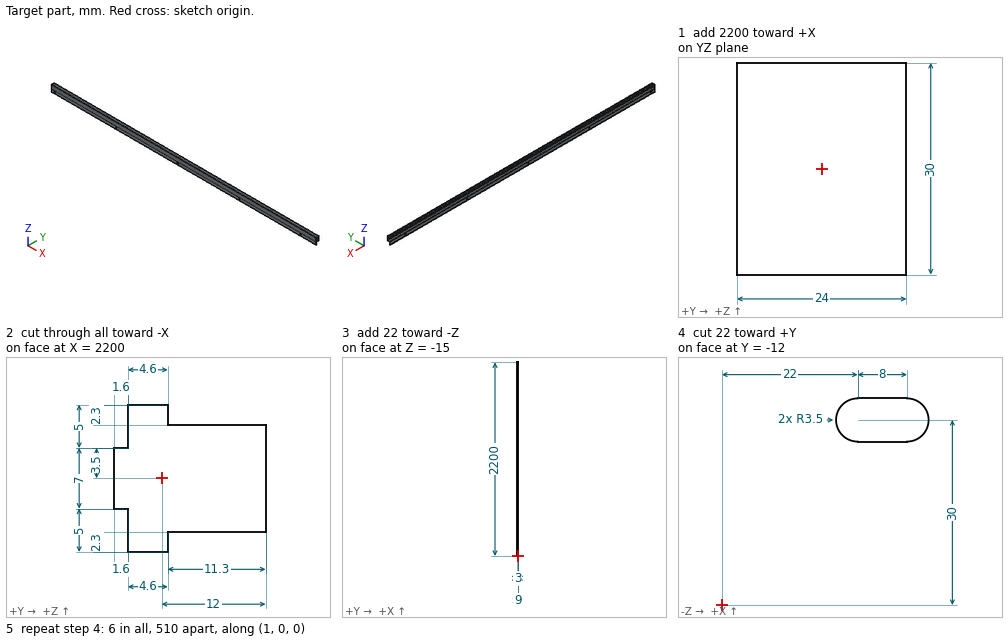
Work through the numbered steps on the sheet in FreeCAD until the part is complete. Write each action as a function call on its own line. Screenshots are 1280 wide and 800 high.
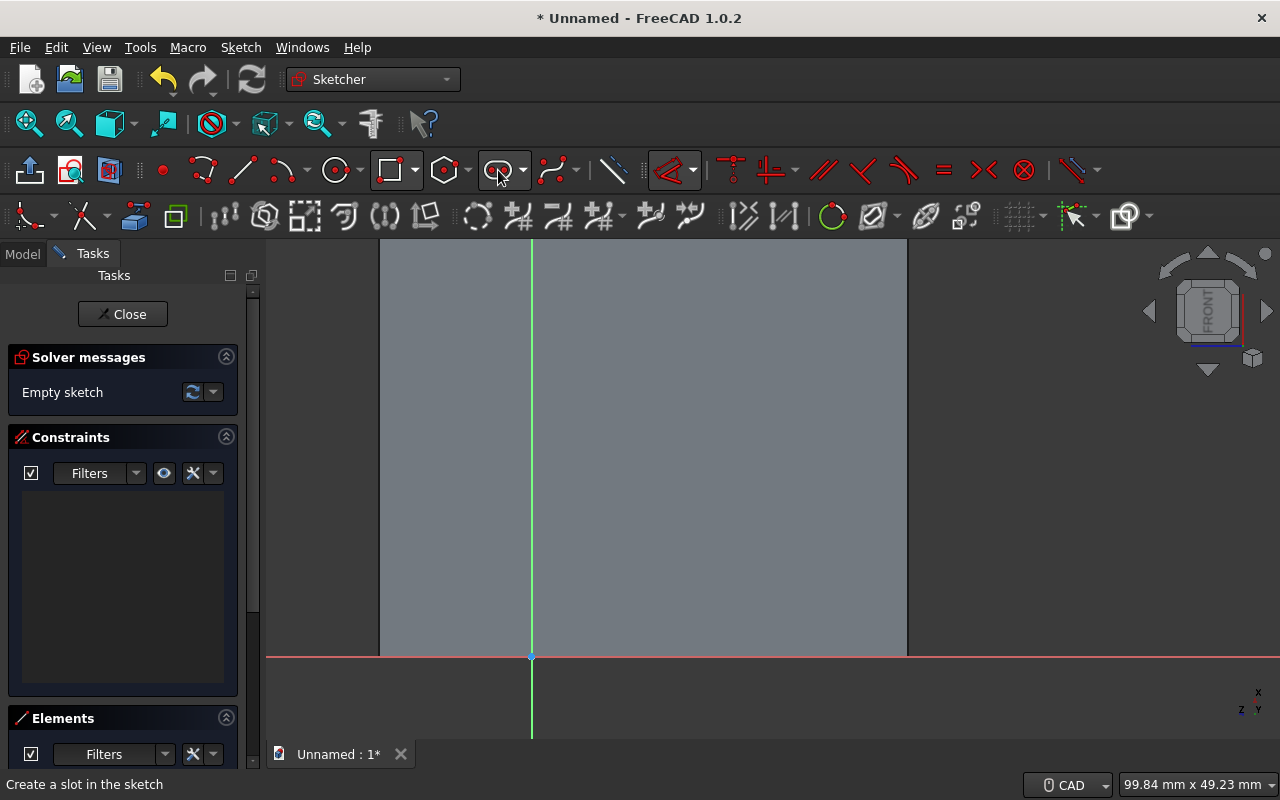
click(755, 352)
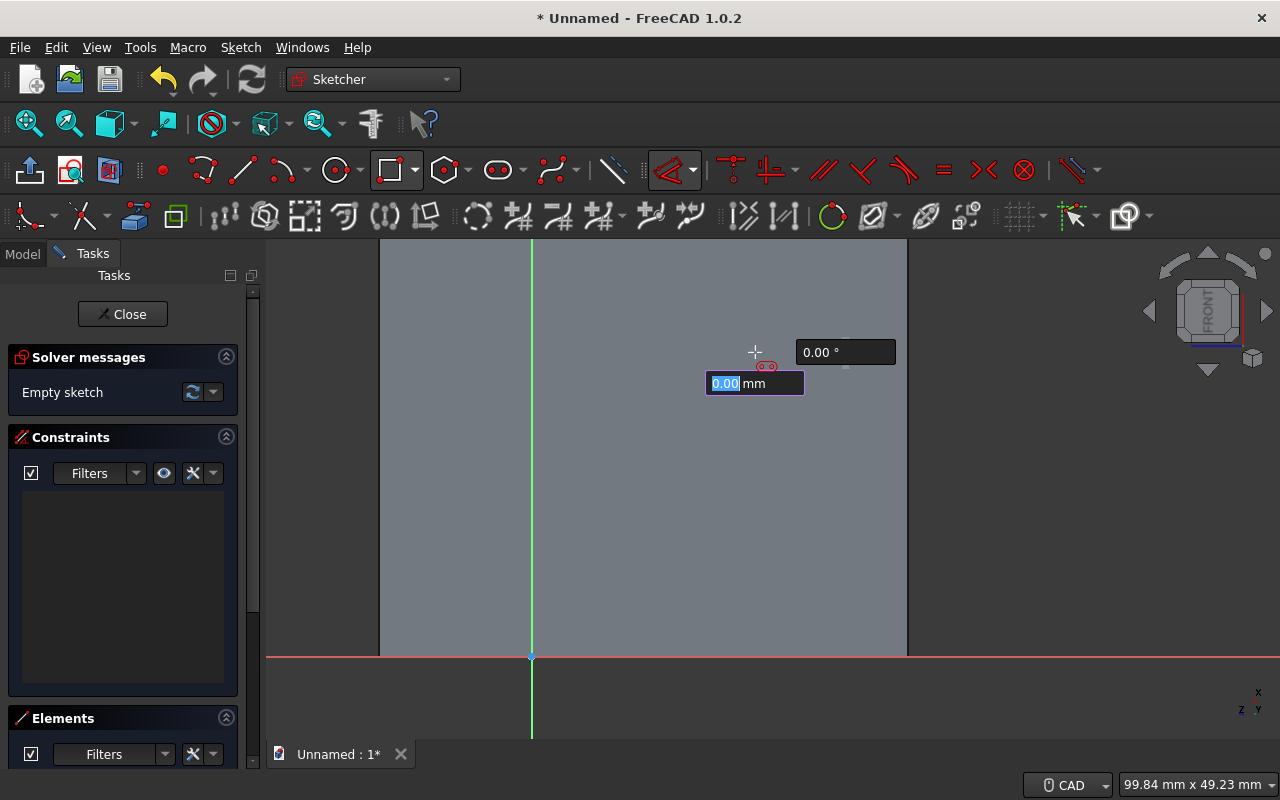
click(836, 352)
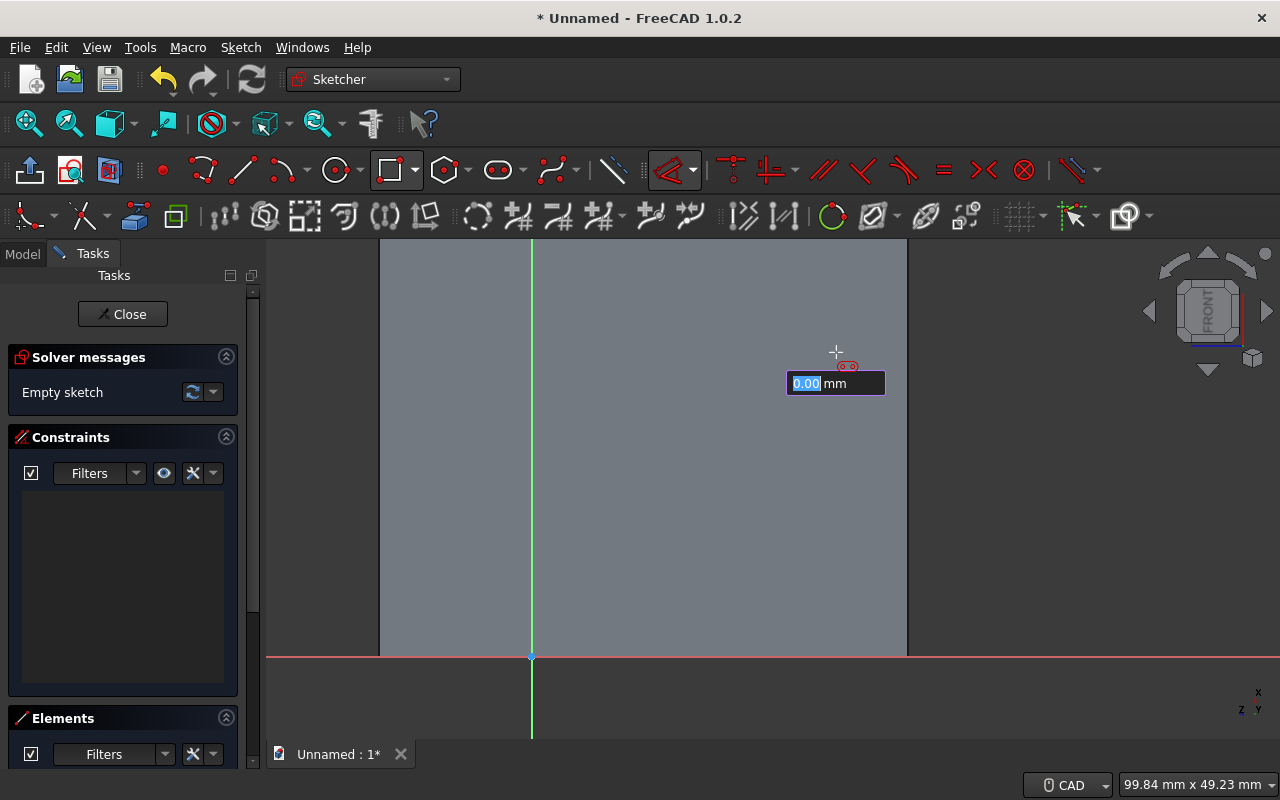
click(796, 317)
key(Escape)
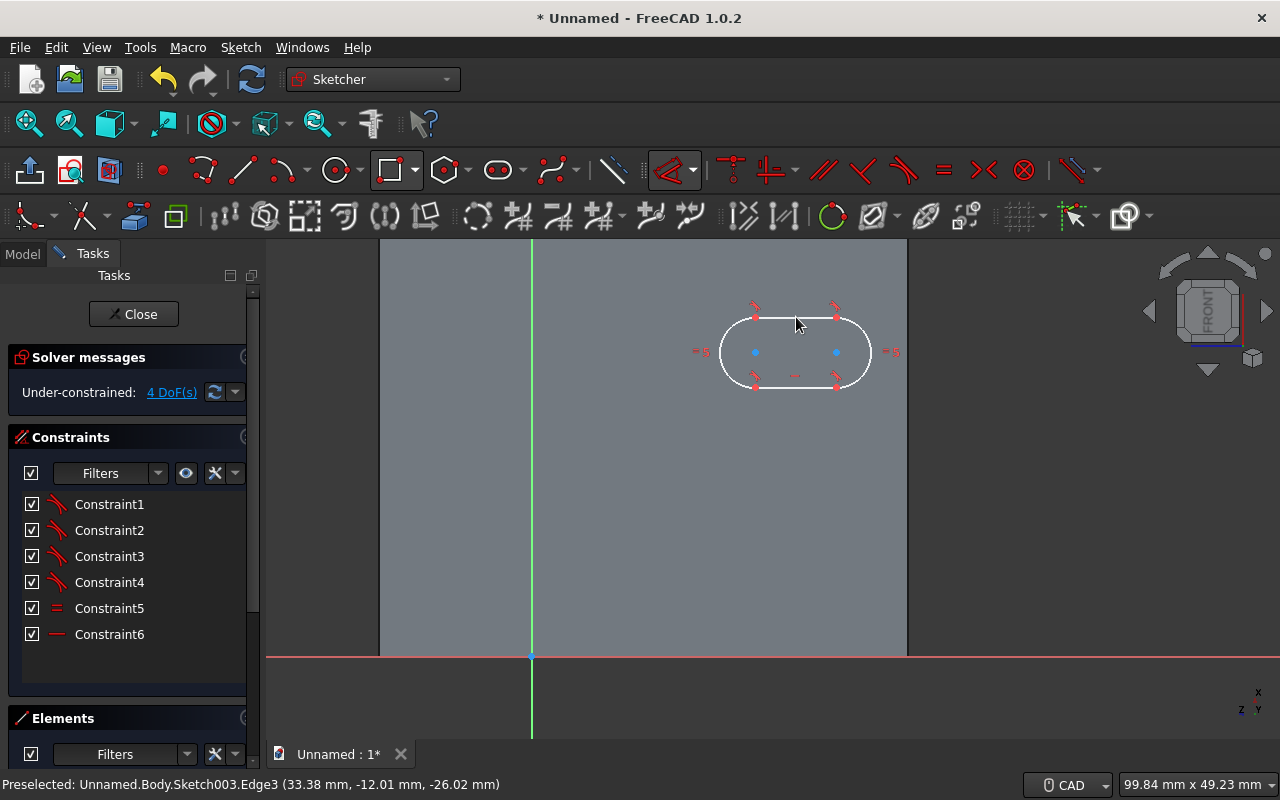
click(727, 332)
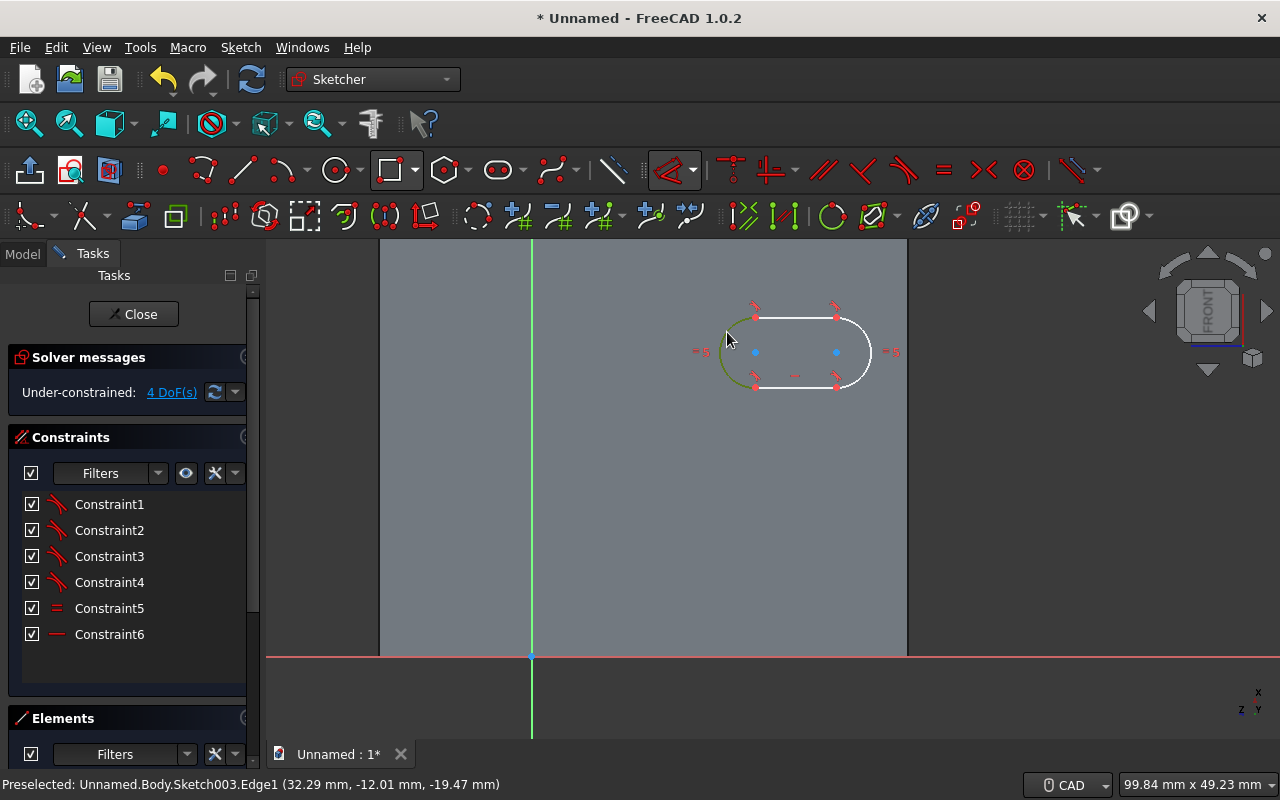
key(k)
key(r)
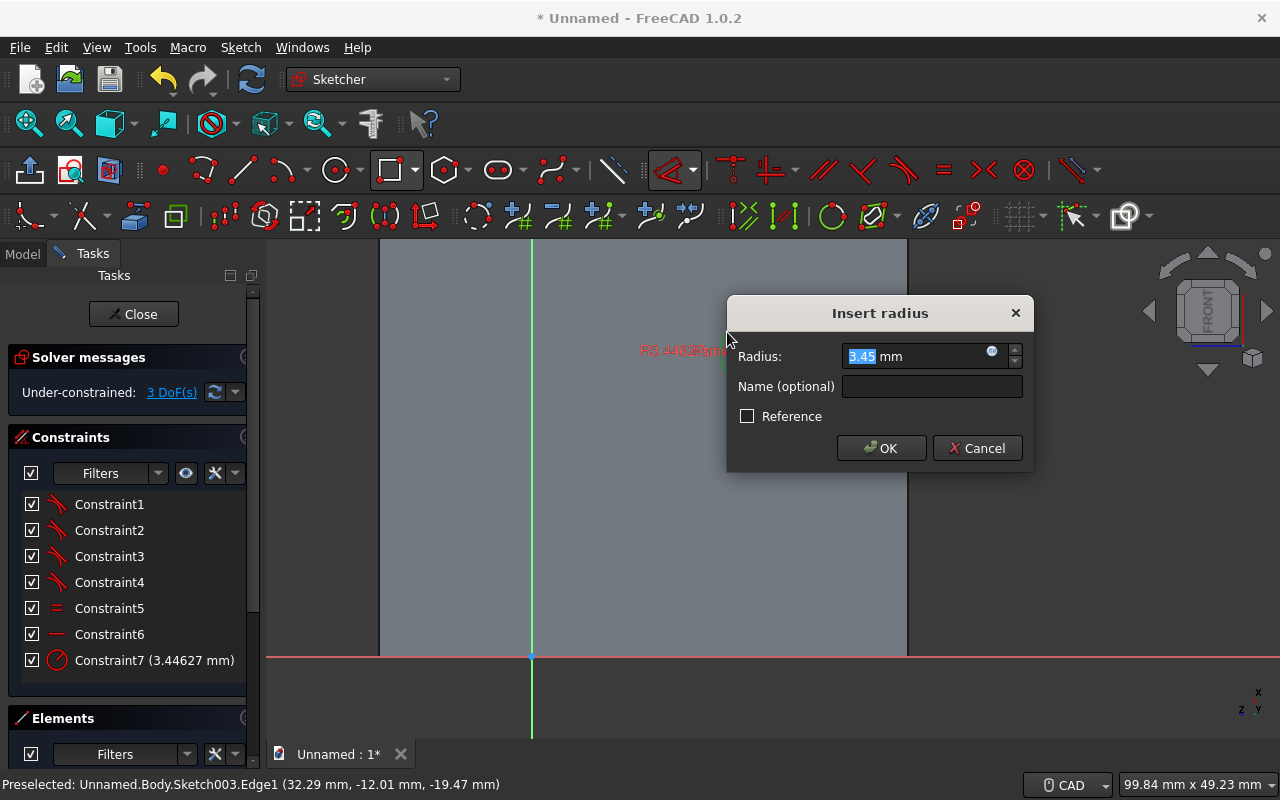
text(3.5)
key(Return)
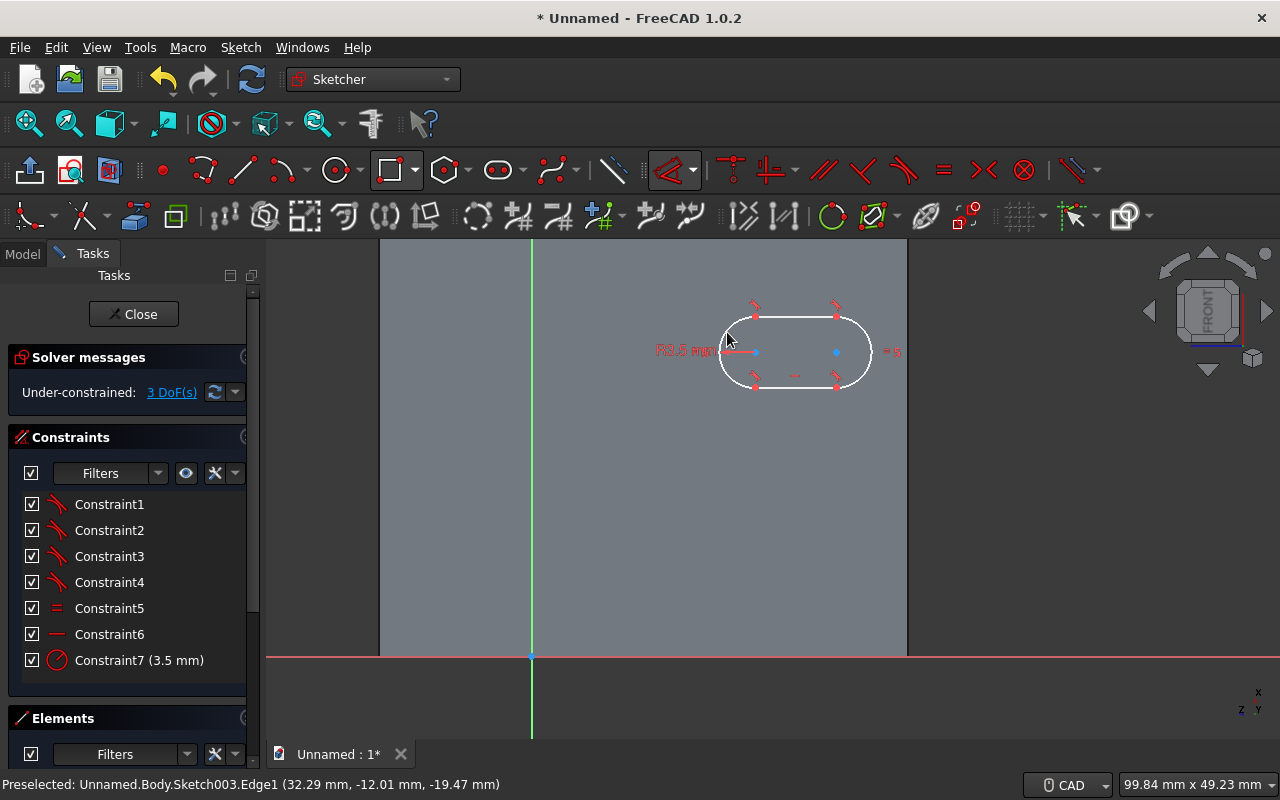
click(779, 317)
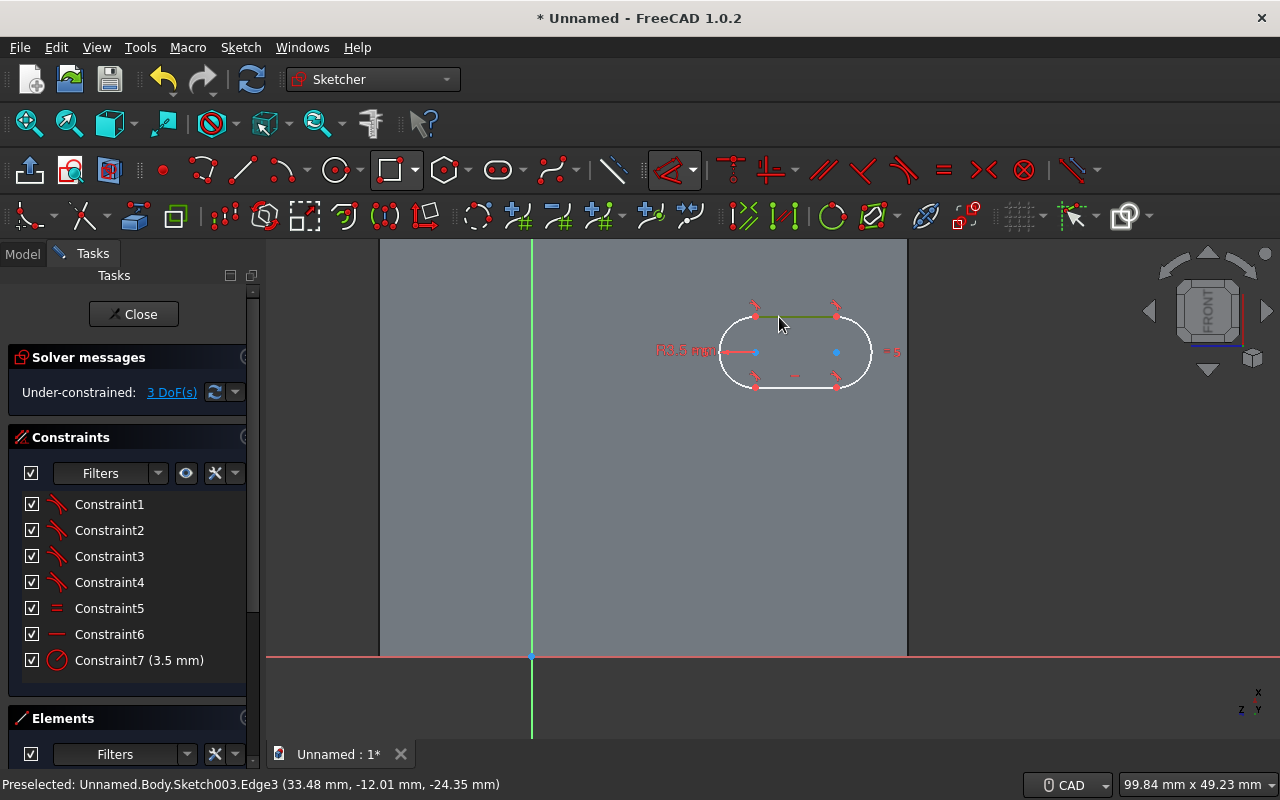
key(l)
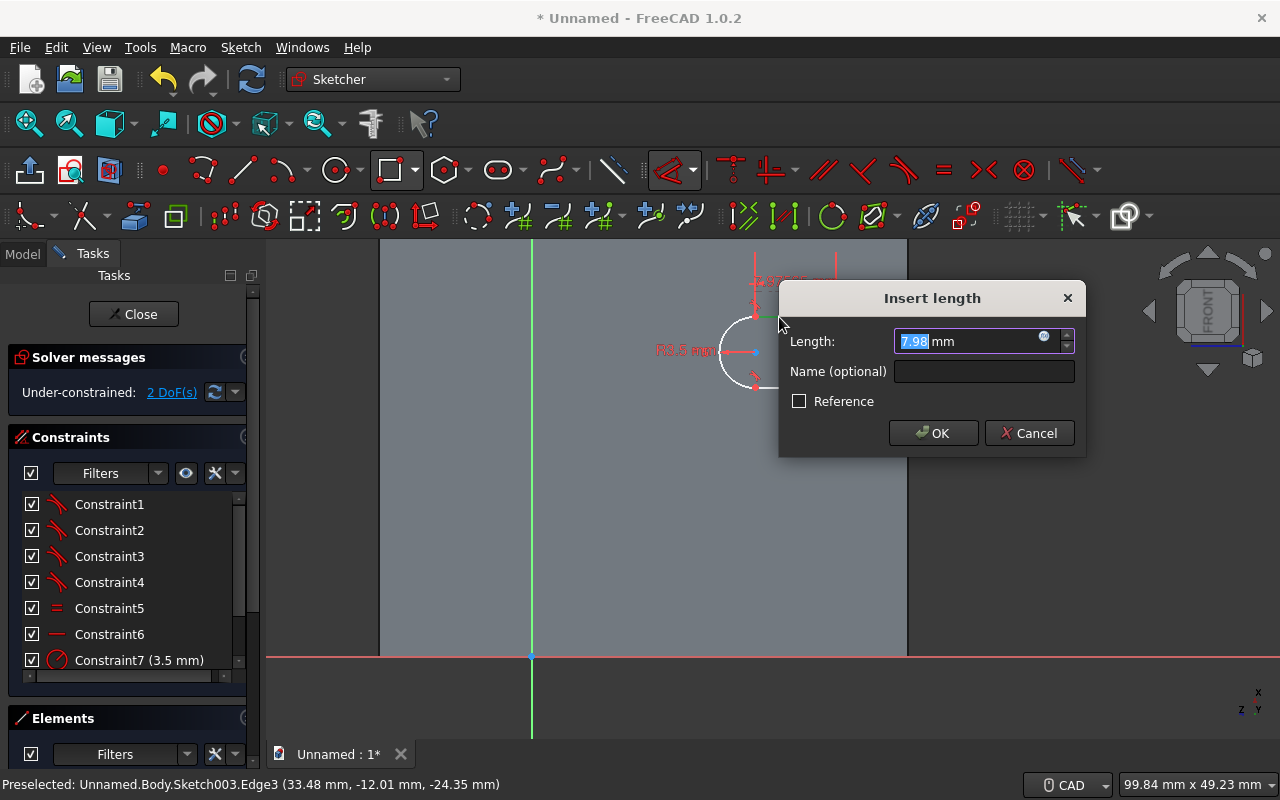
text(8)
key(Return)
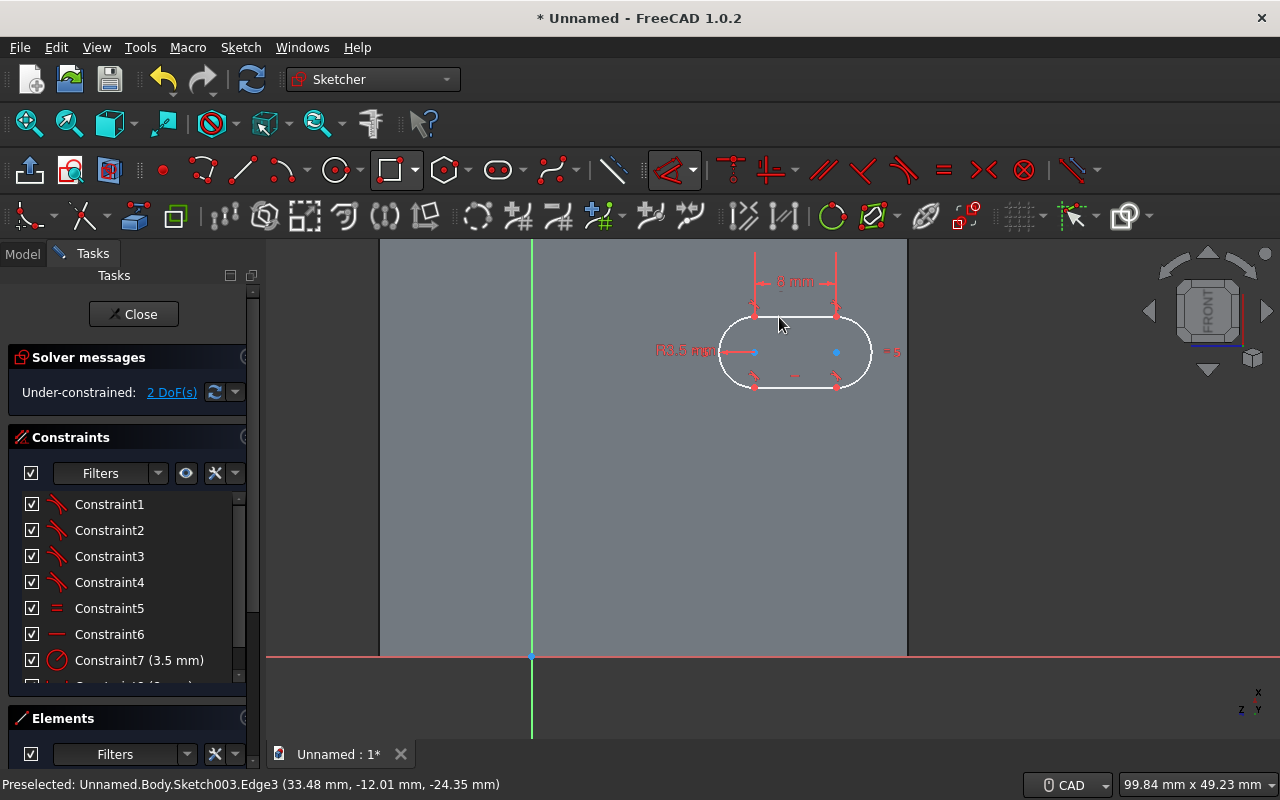
click(755, 317)